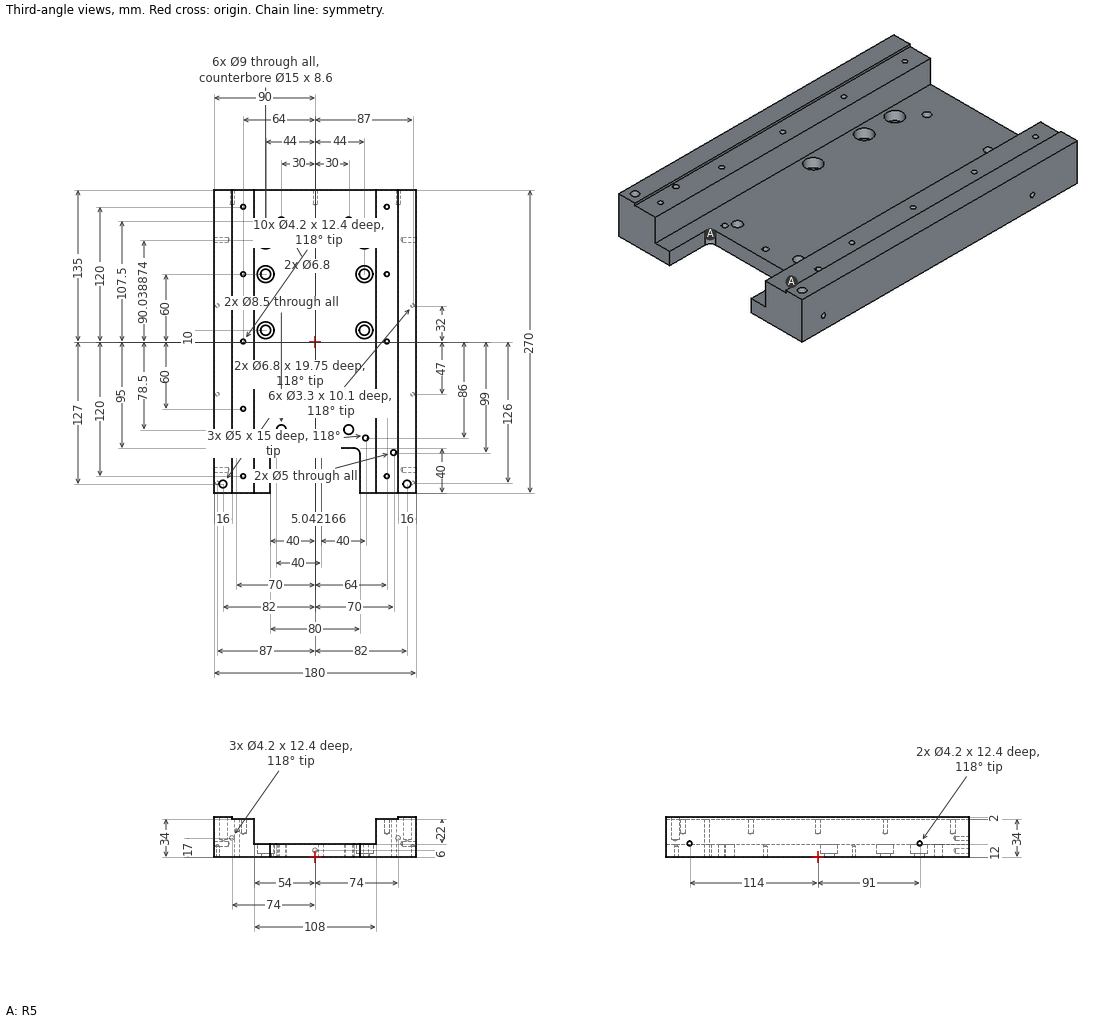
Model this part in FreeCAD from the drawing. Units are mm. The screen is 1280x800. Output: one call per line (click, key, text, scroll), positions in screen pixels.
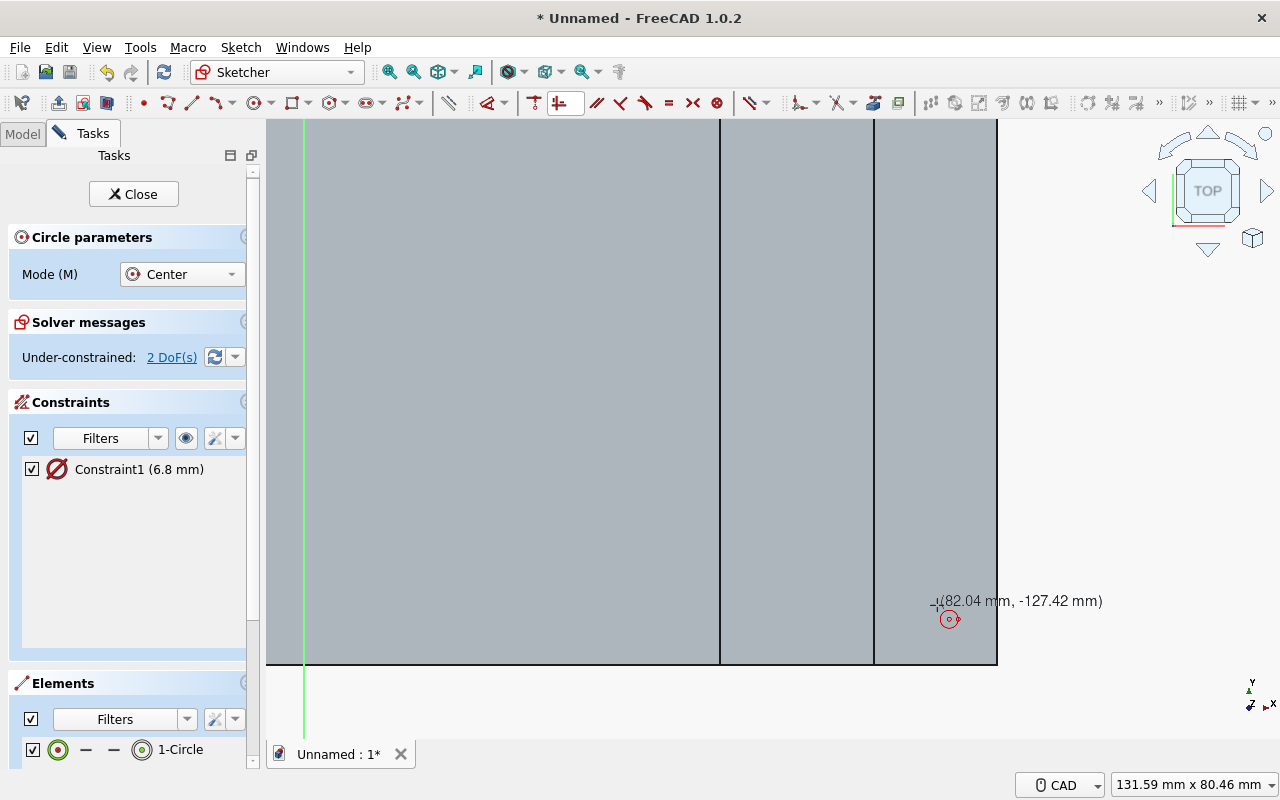
click(936, 603)
move(954, 585)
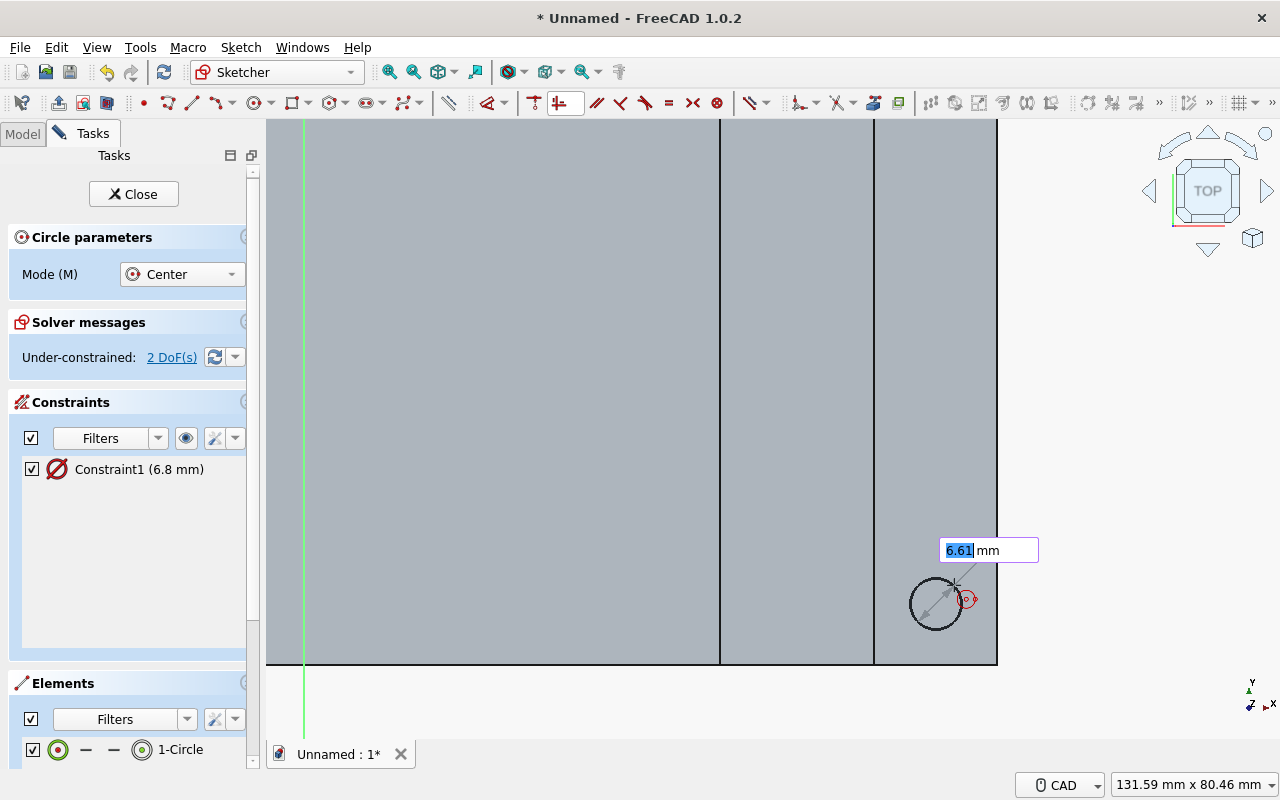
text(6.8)
key(Return)
key(Escape)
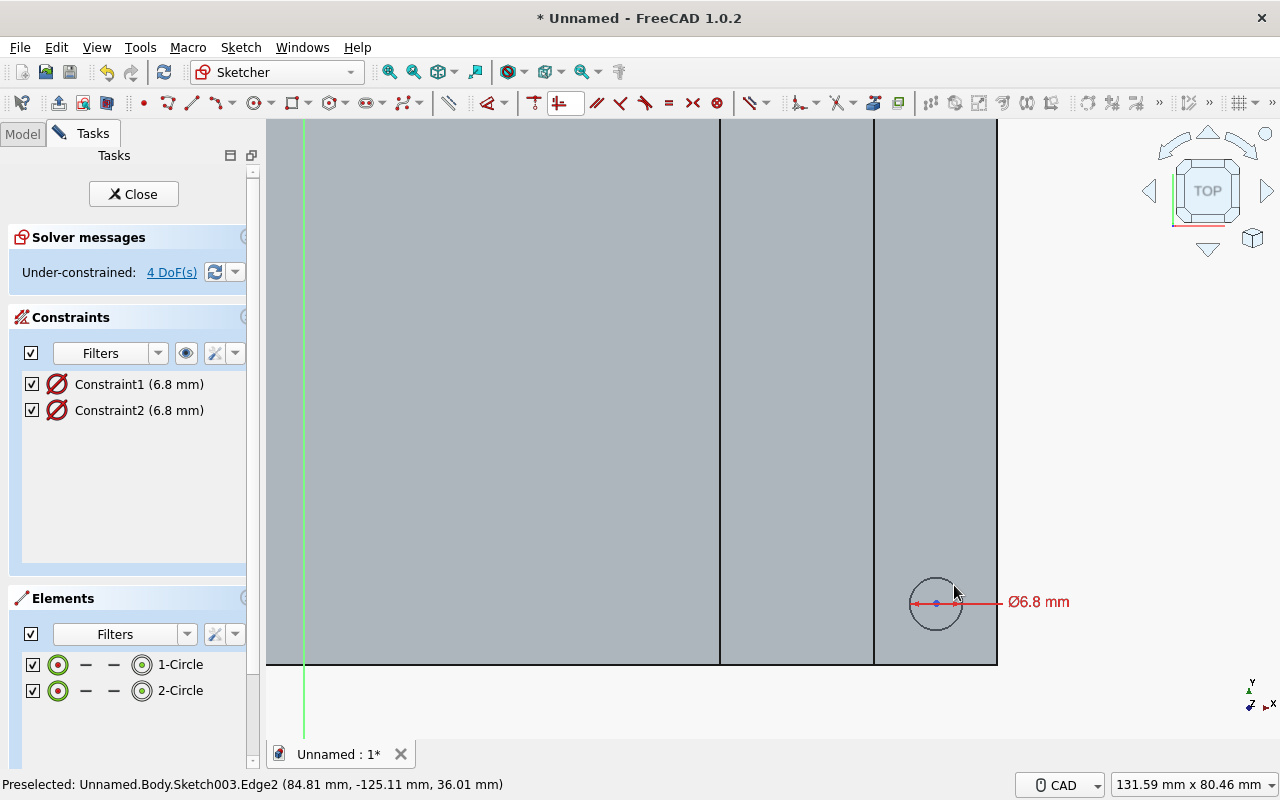
scroll(938, 605, down, 5)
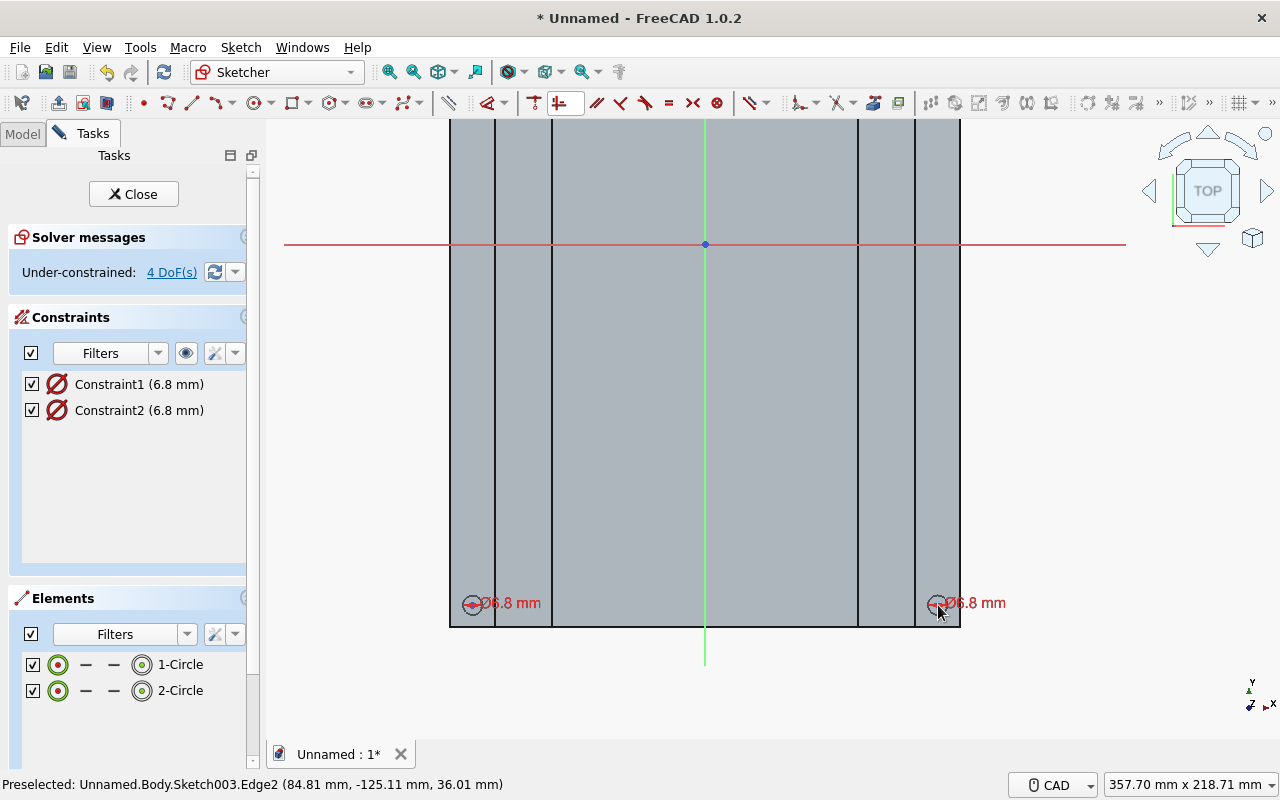
click(473, 605)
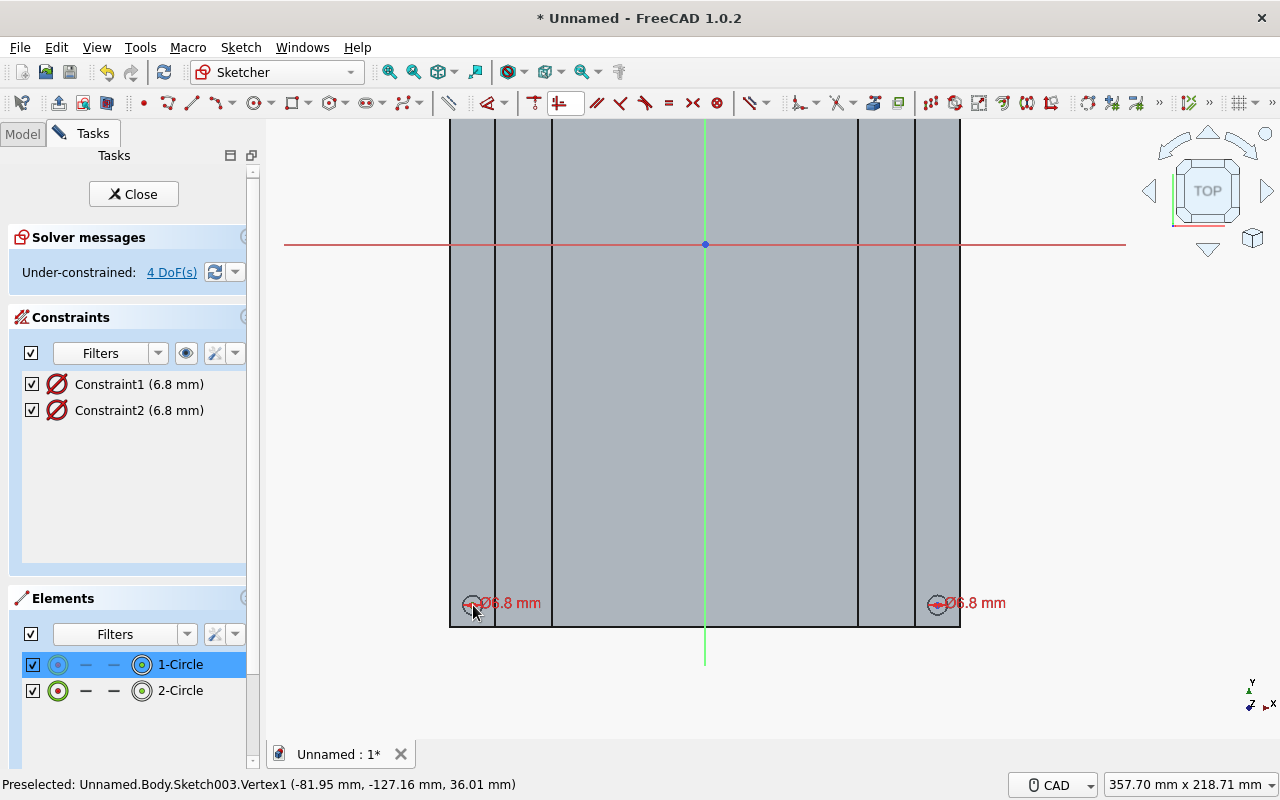
click(938, 605)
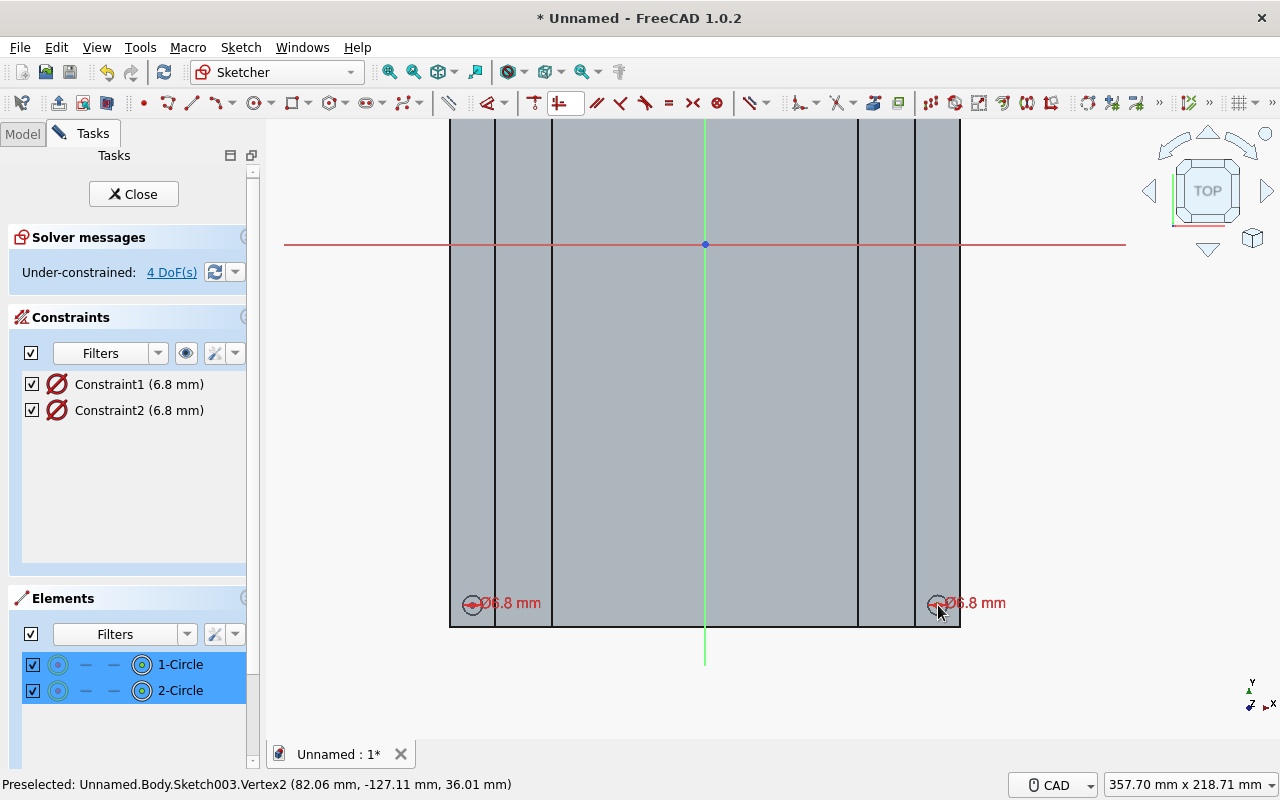
click(578, 104)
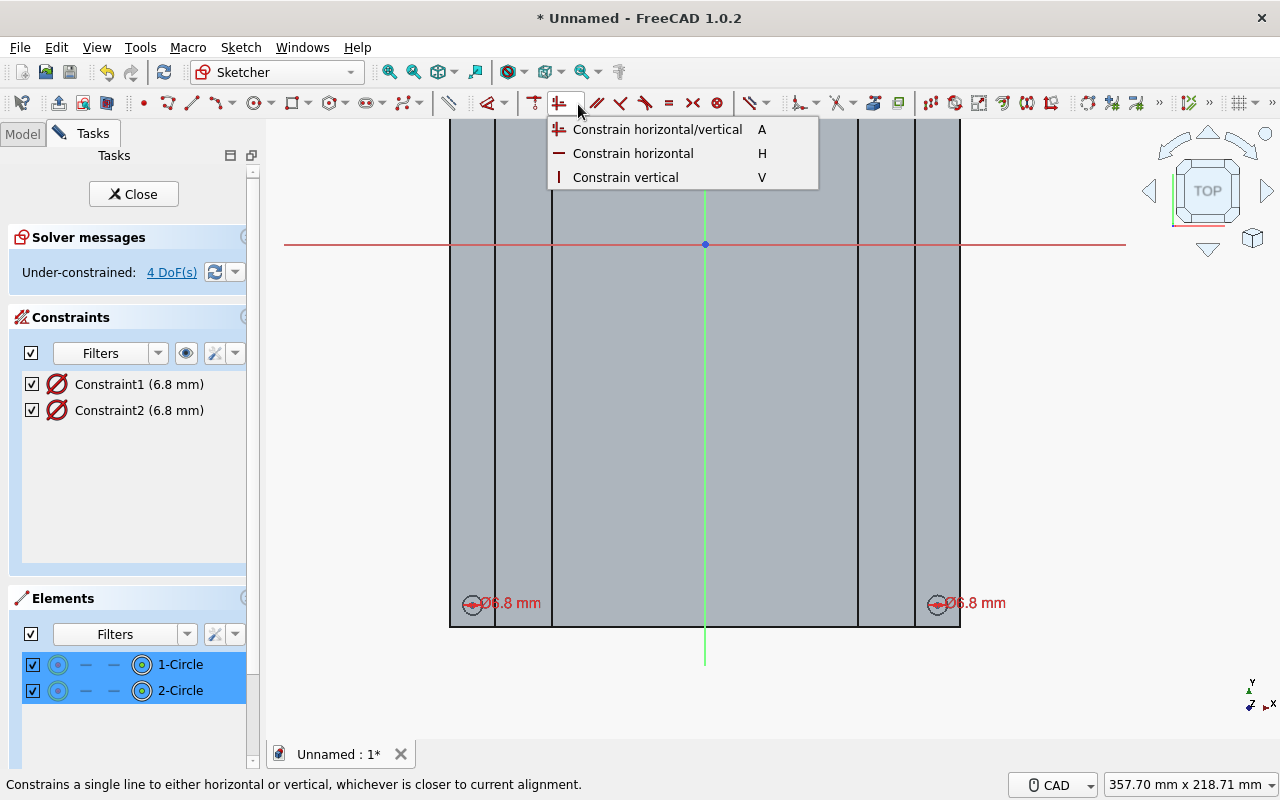
click(683, 153)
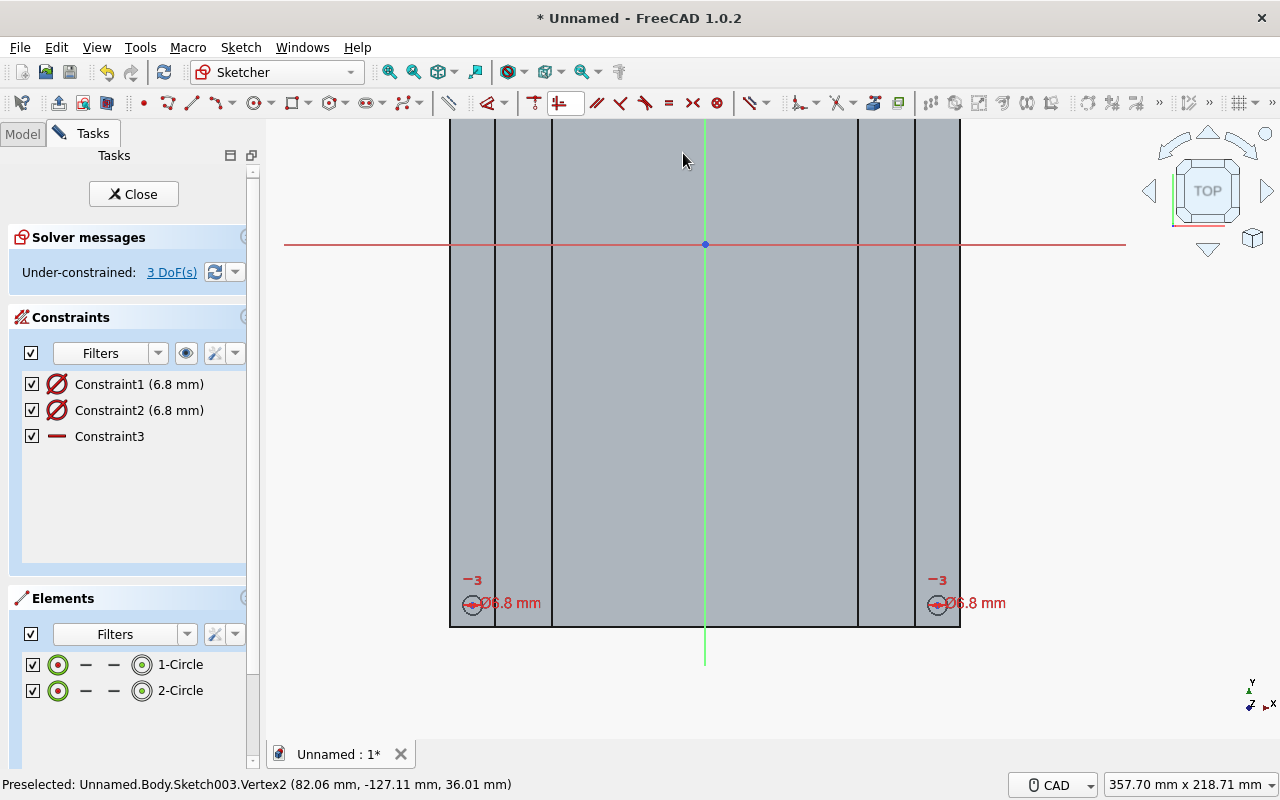
key(d)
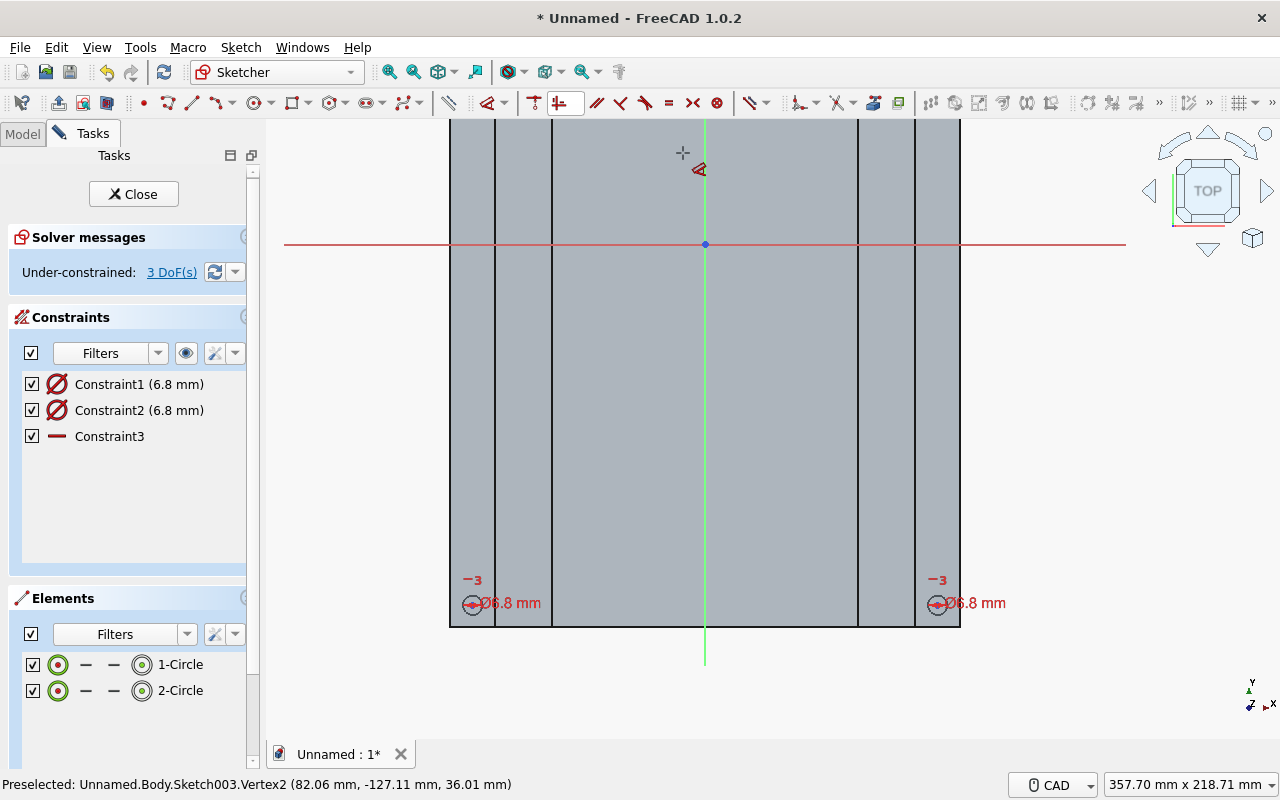
click(473, 605)
click(589, 211)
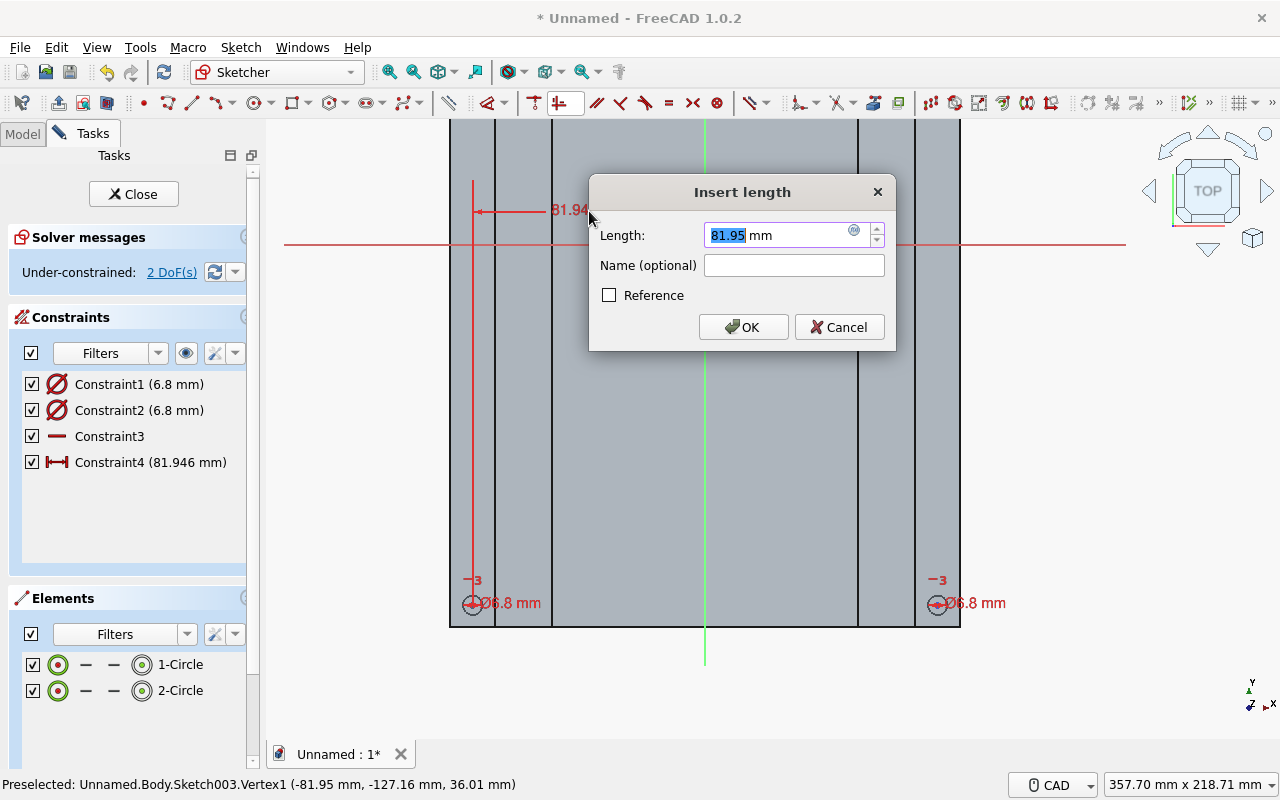
text(82)
key(Return)